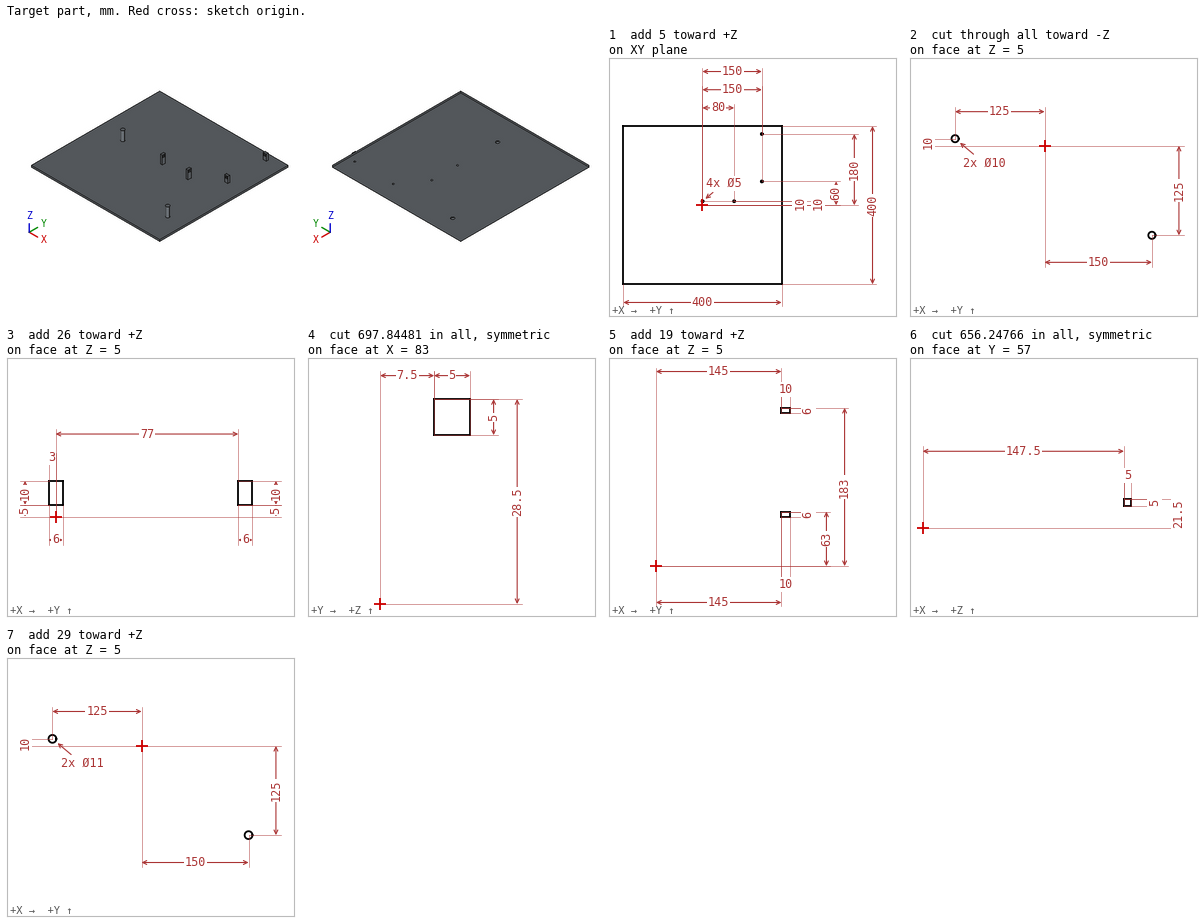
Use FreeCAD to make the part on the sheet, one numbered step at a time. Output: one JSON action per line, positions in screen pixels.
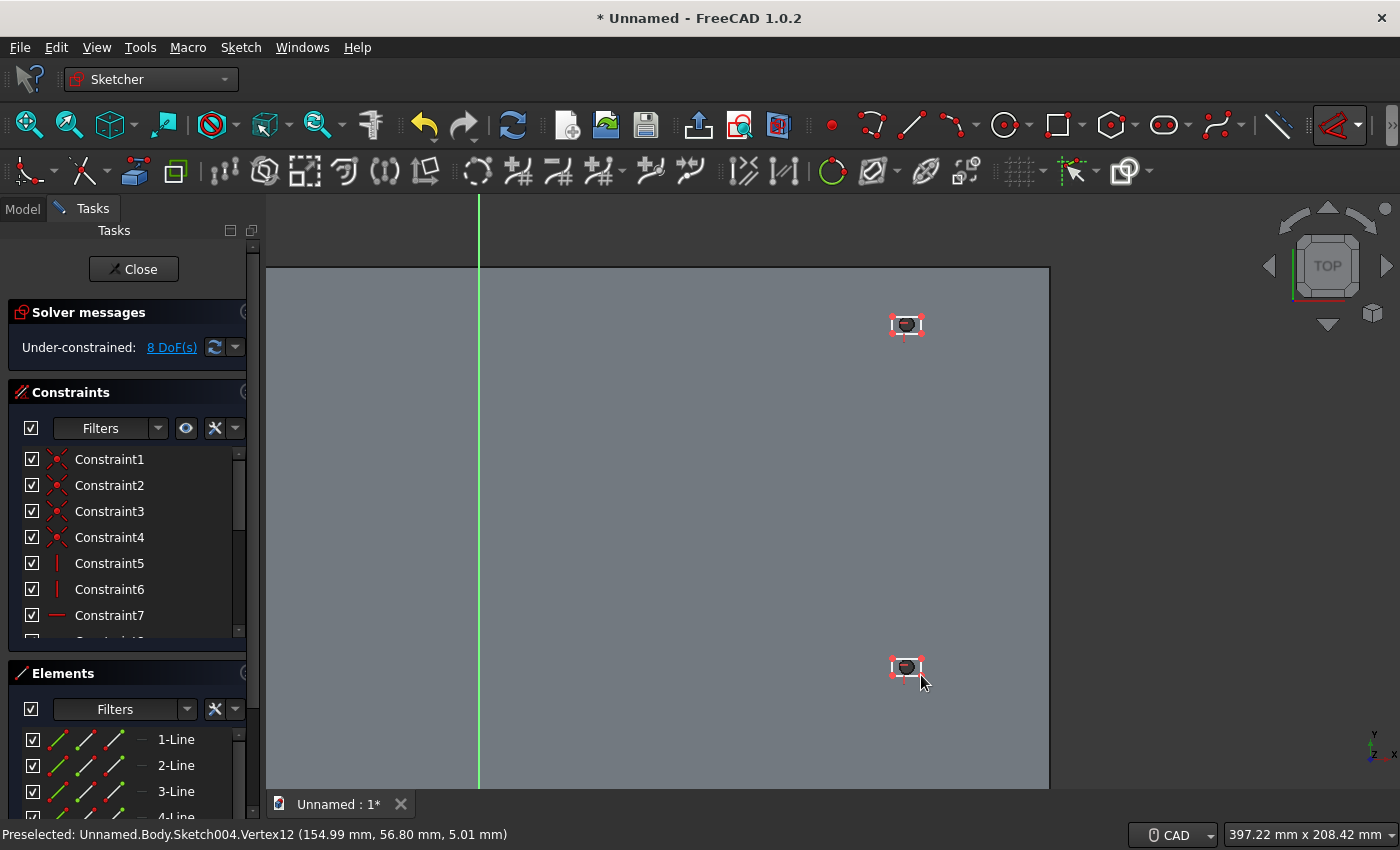
{"action": "scroll", "coordinate": [892, 325], "scroll_direction": "up", "scroll_amount": 5}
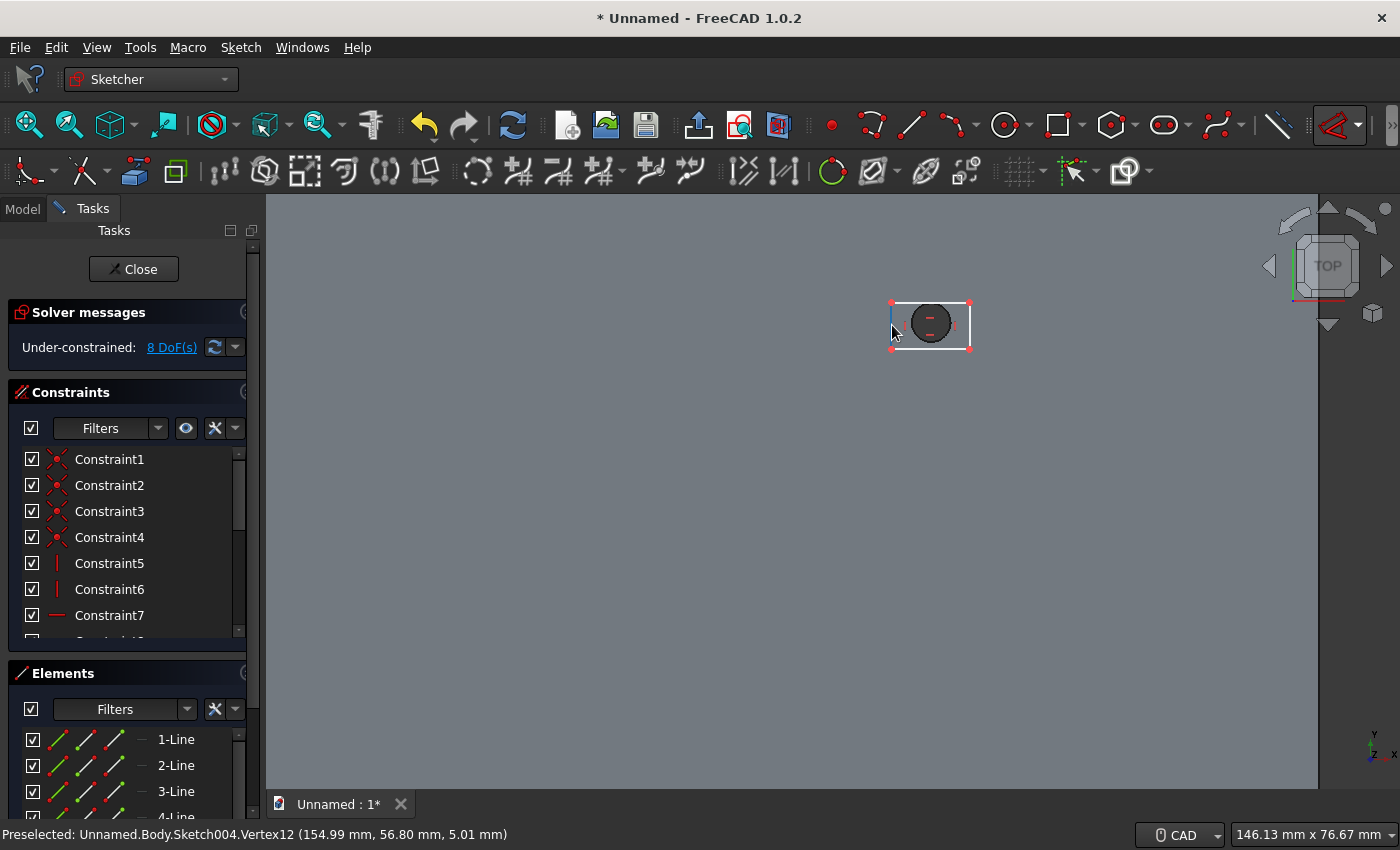
{"action": "left_click", "coordinate": [891, 326]}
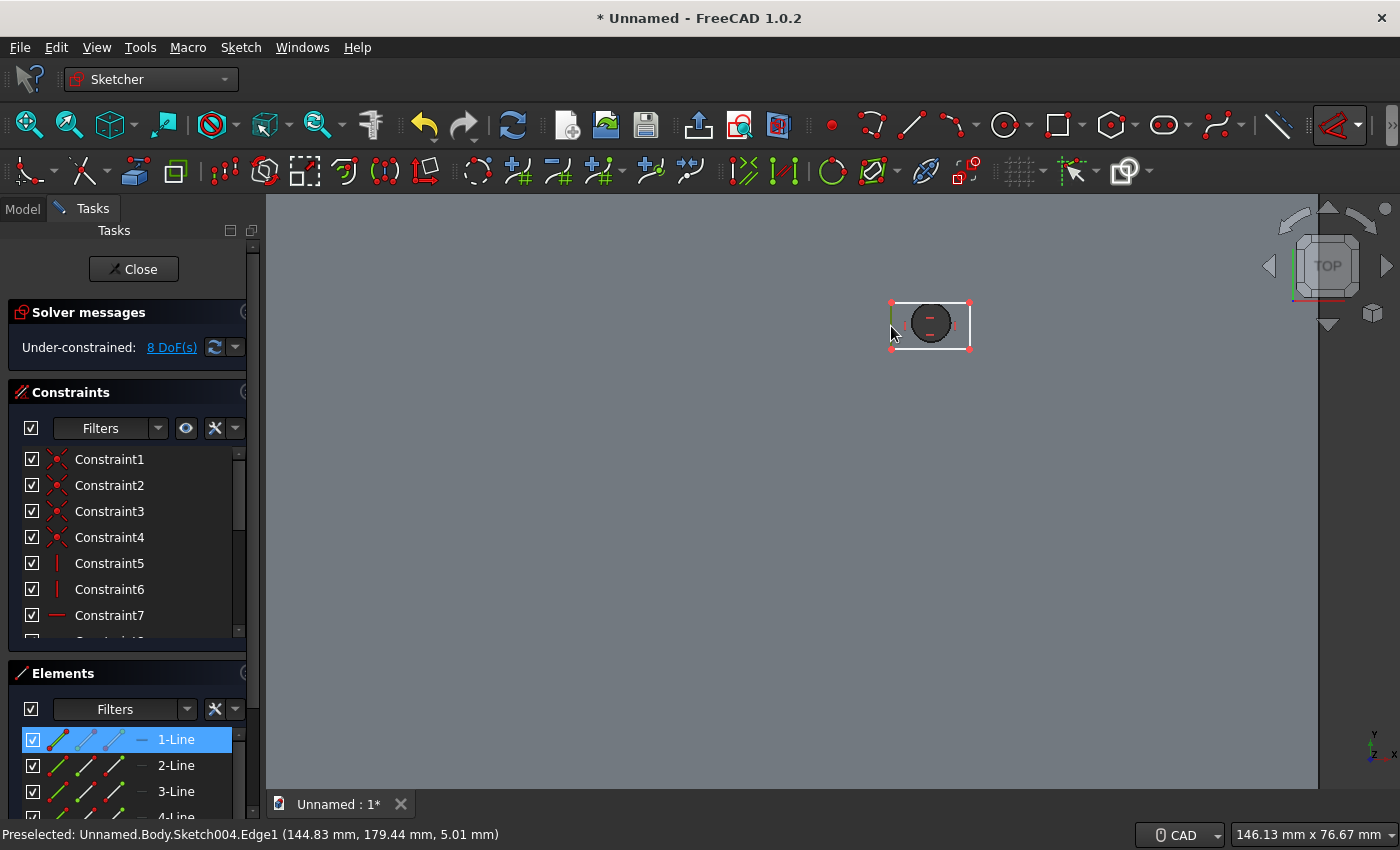
{"action": "key", "text": "i"}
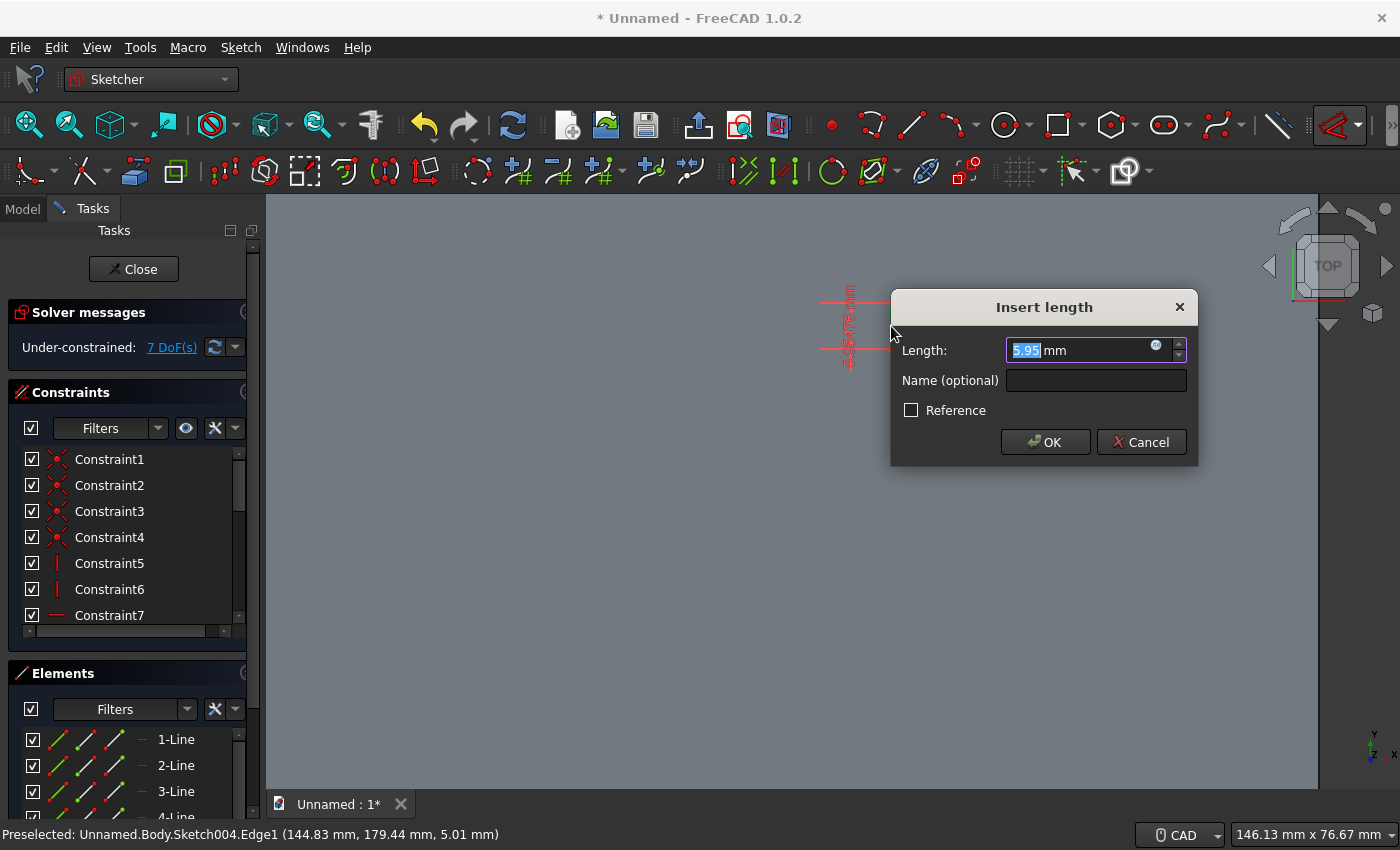
{"action": "type", "text": "6"}
{"action": "key", "text": "Return"}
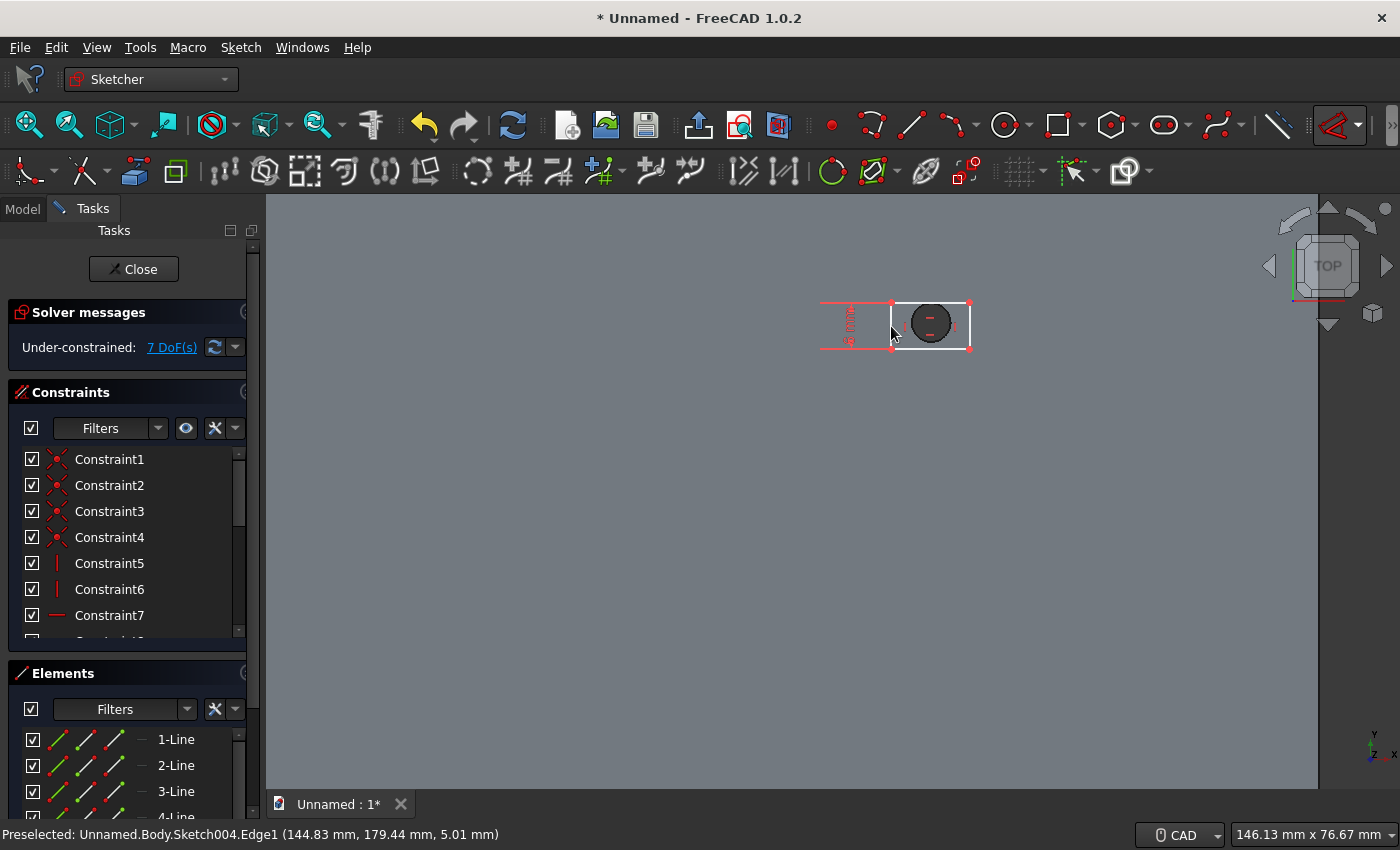
{"action": "scroll", "coordinate": [894, 322], "scroll_direction": "down", "scroll_amount": 7}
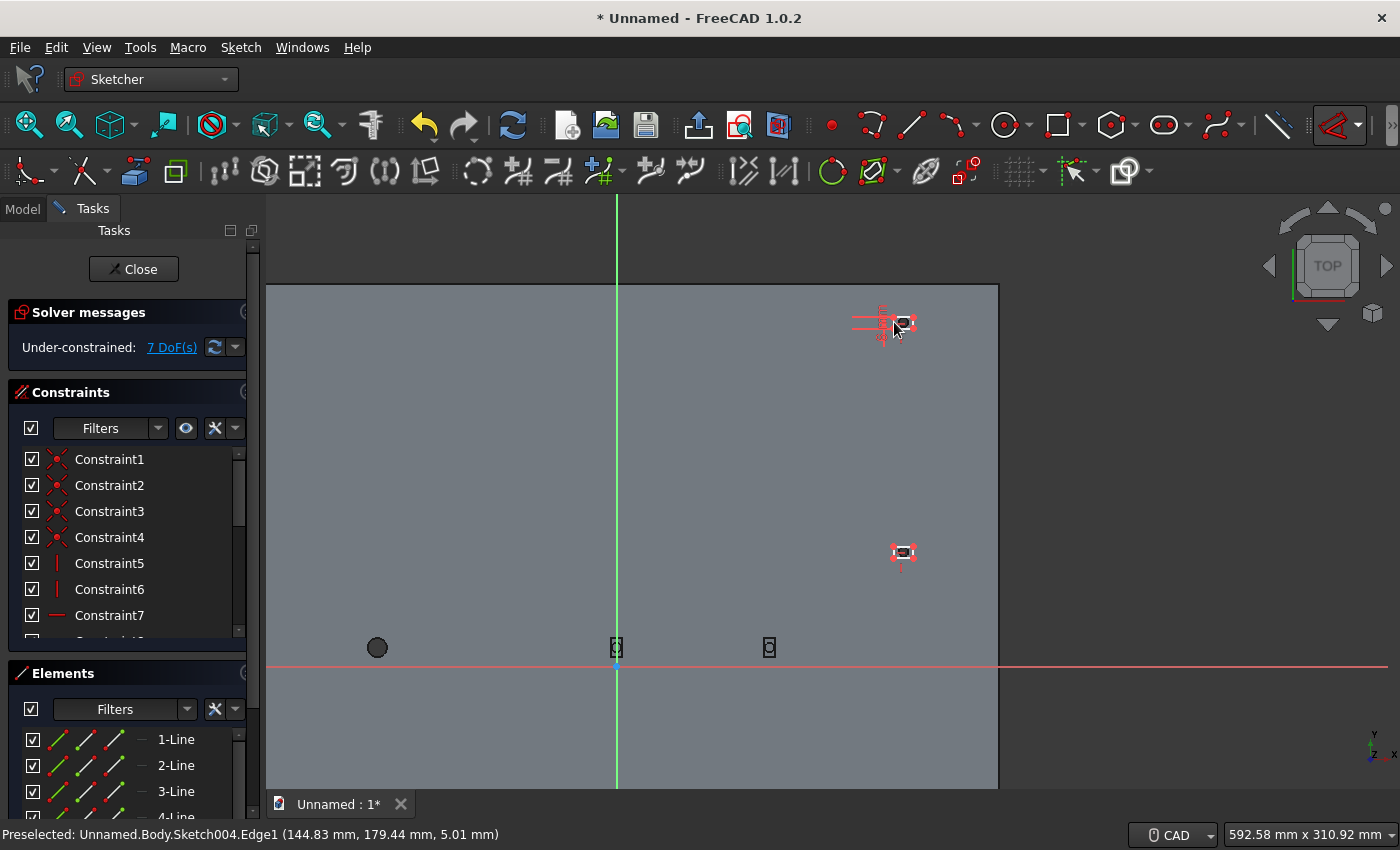
{"action": "scroll", "coordinate": [894, 550], "scroll_direction": "up", "scroll_amount": 7}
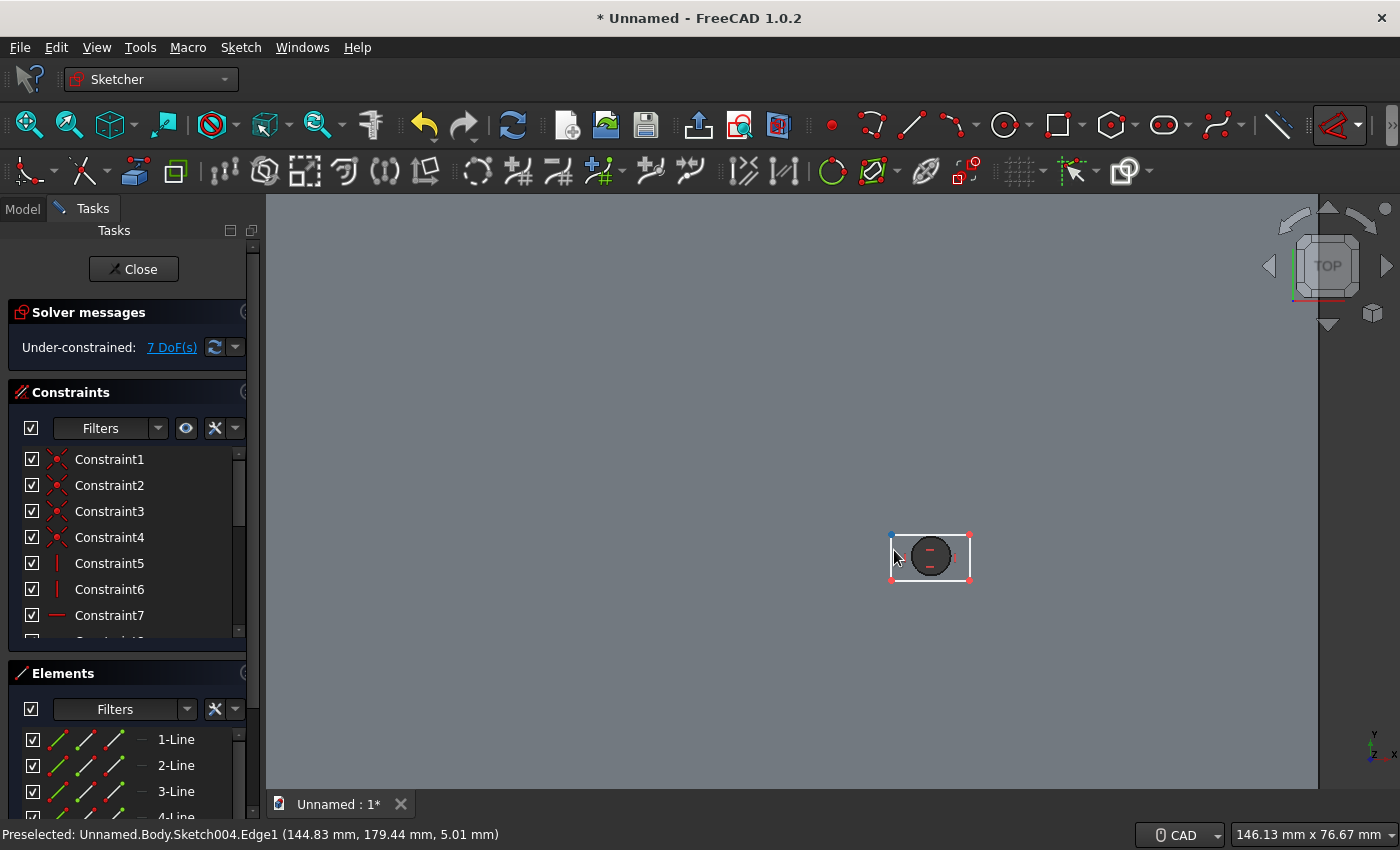
{"action": "left_click", "coordinate": [891, 549]}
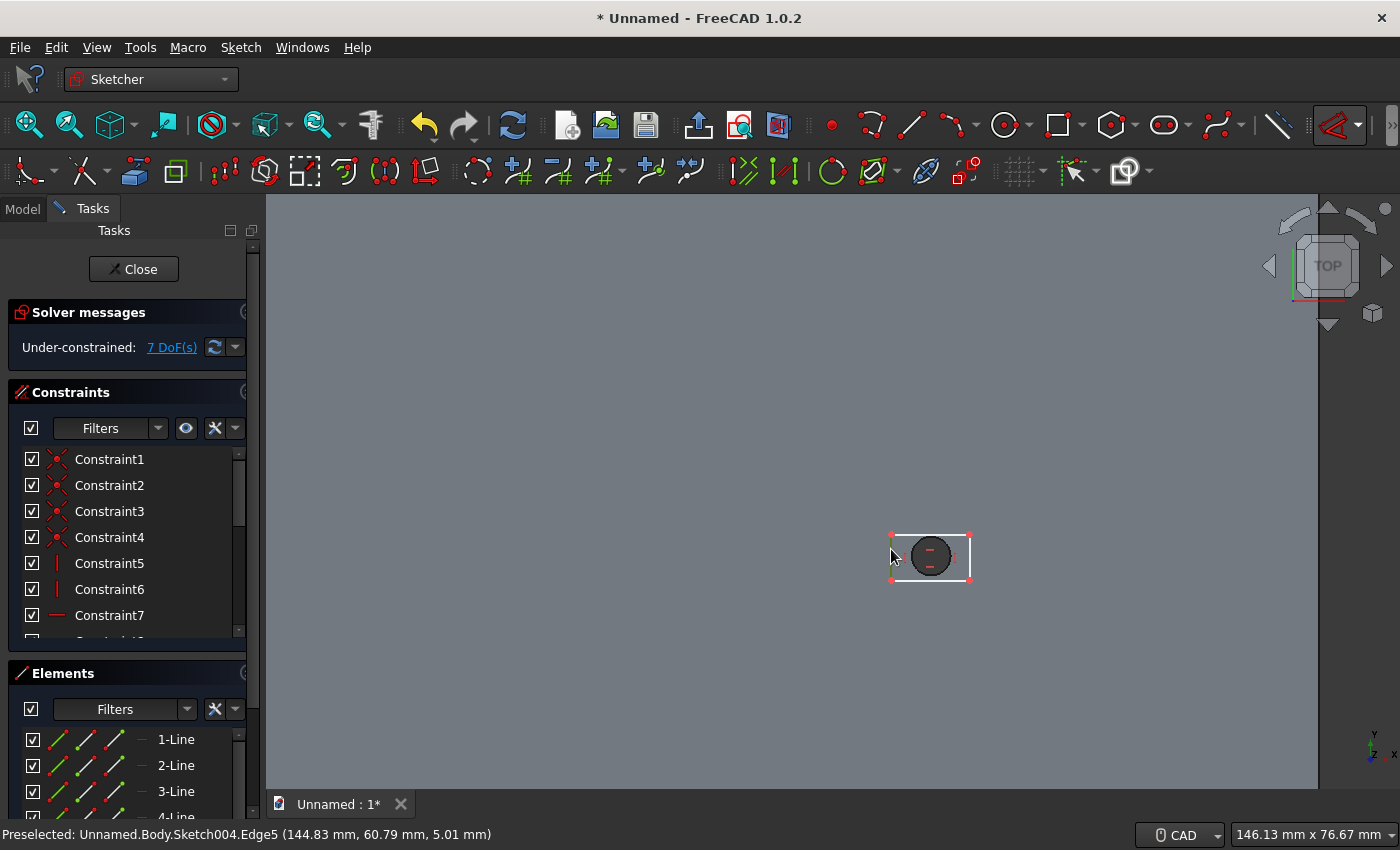
{"action": "key", "text": "i"}